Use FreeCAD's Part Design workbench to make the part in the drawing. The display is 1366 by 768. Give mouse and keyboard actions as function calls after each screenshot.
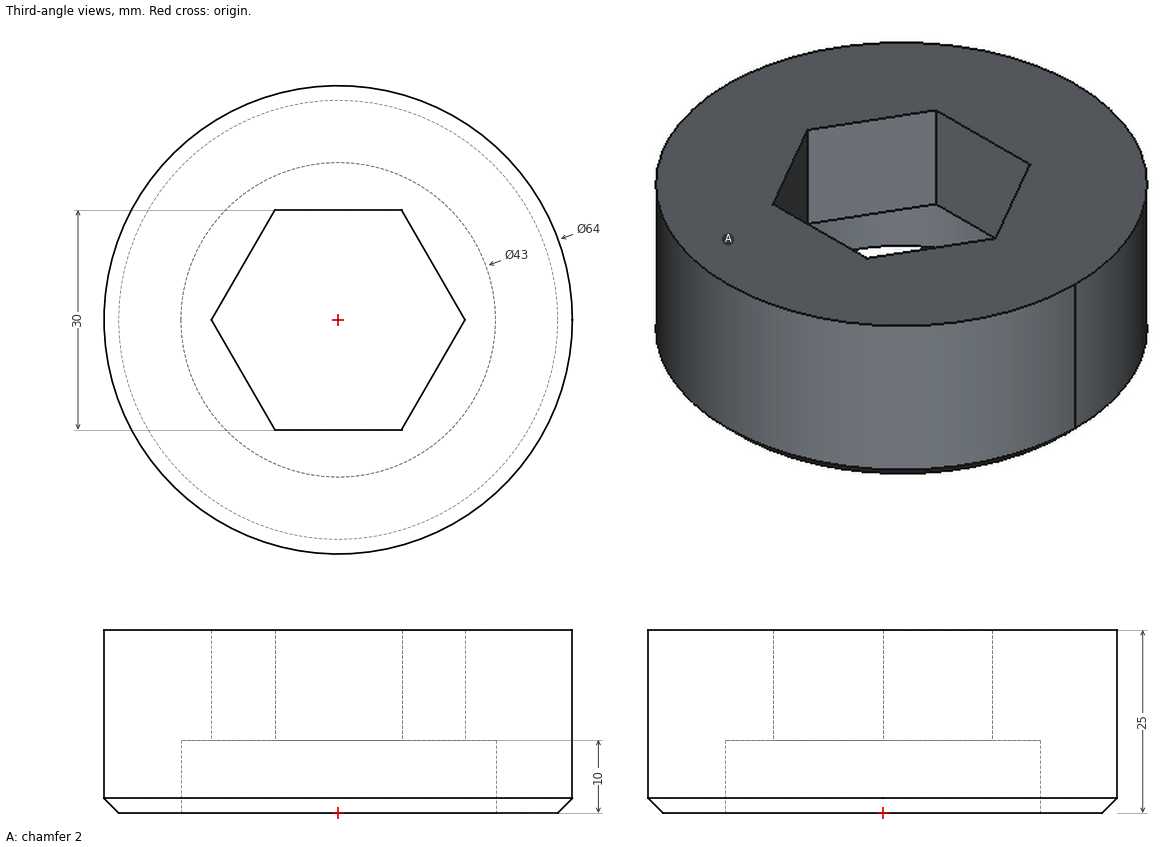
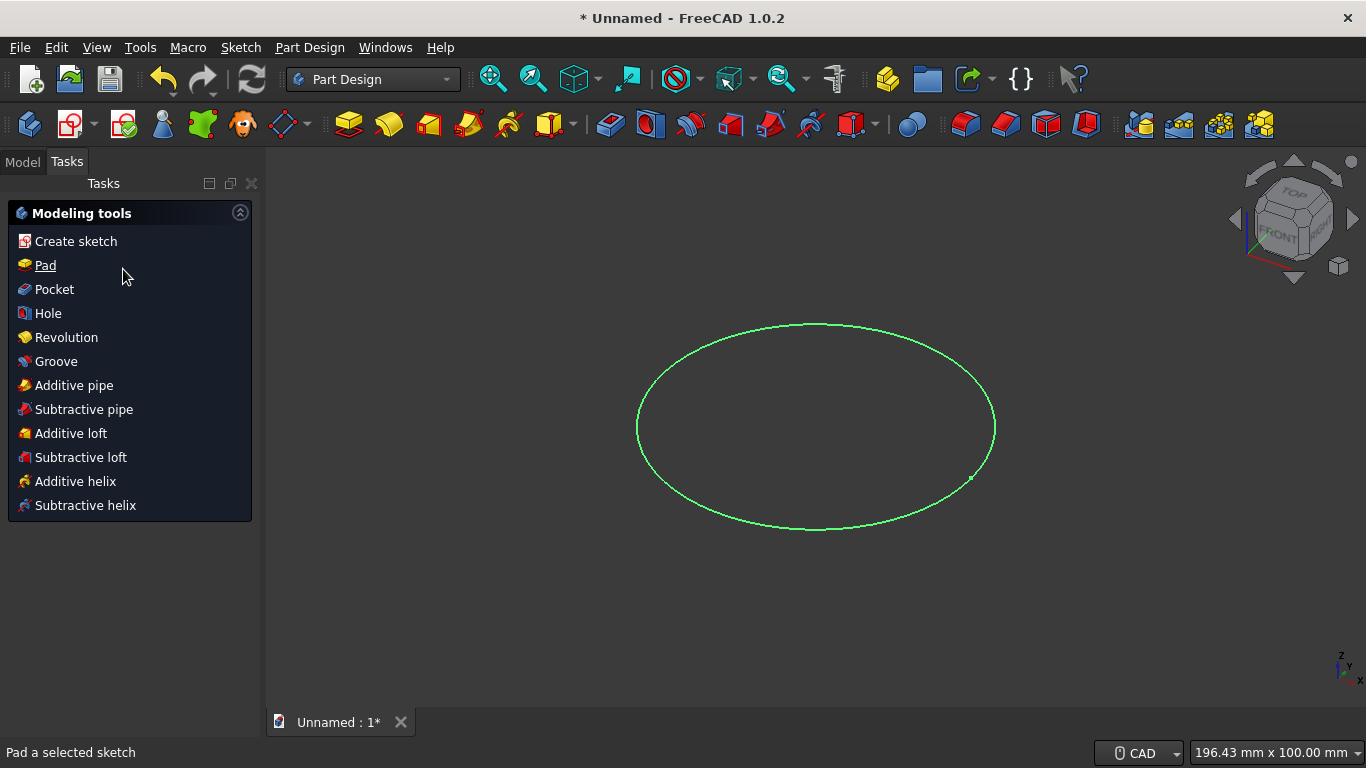
click(350, 124)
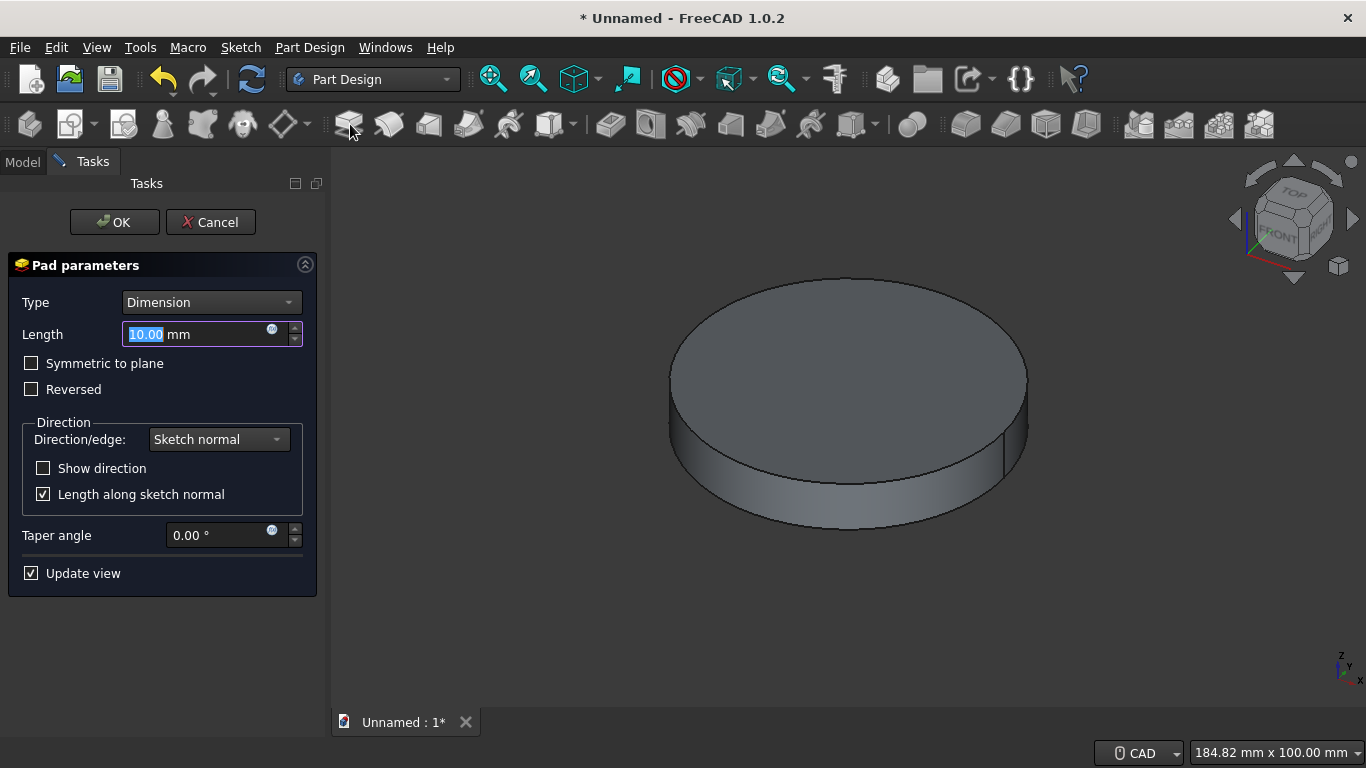
text(25)
key(Tab)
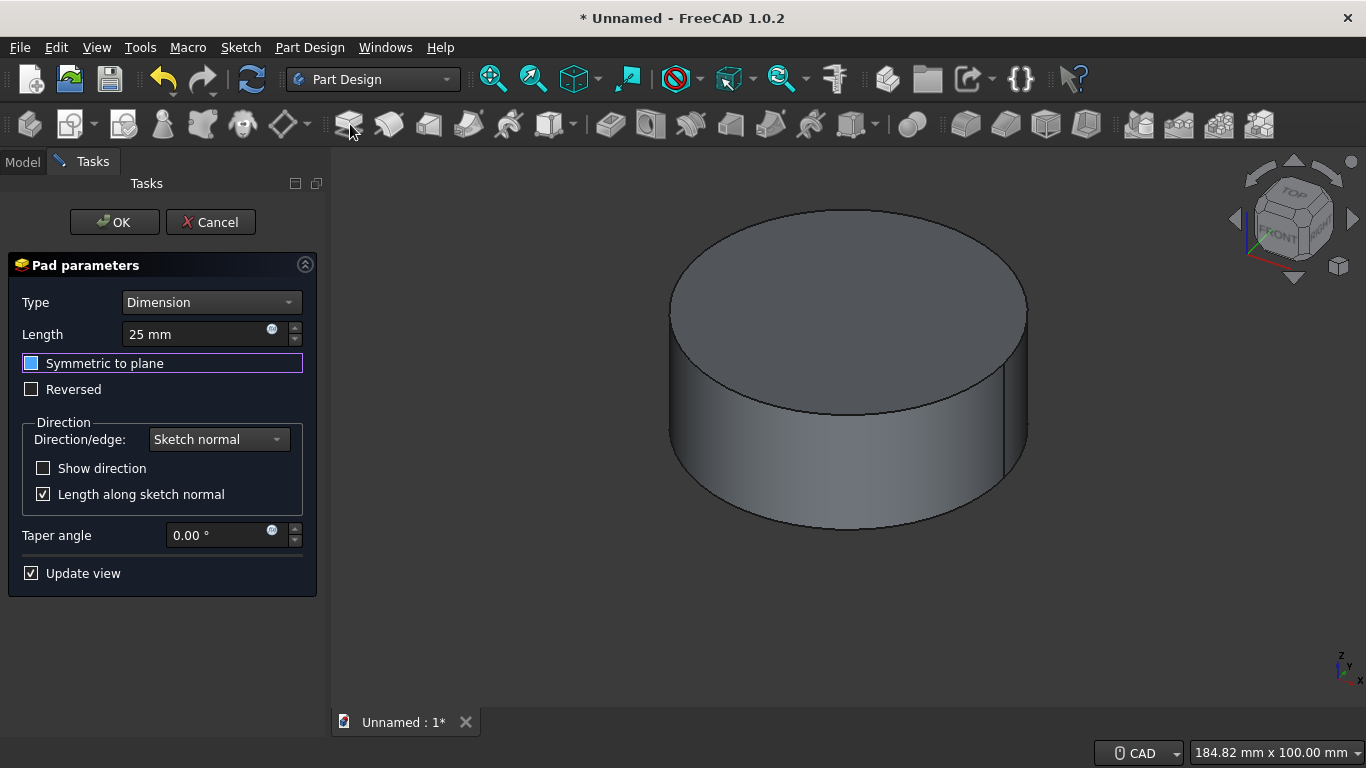
click(115, 222)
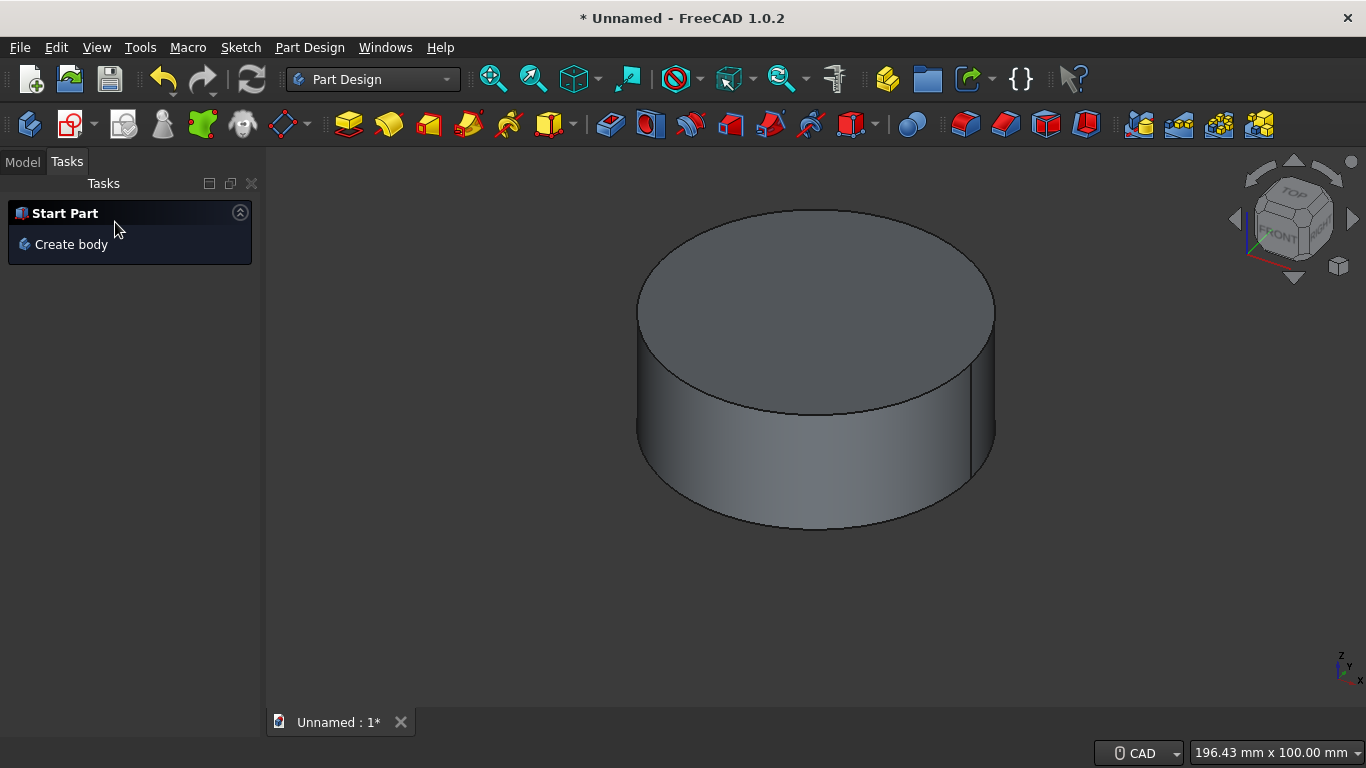
click(816, 311)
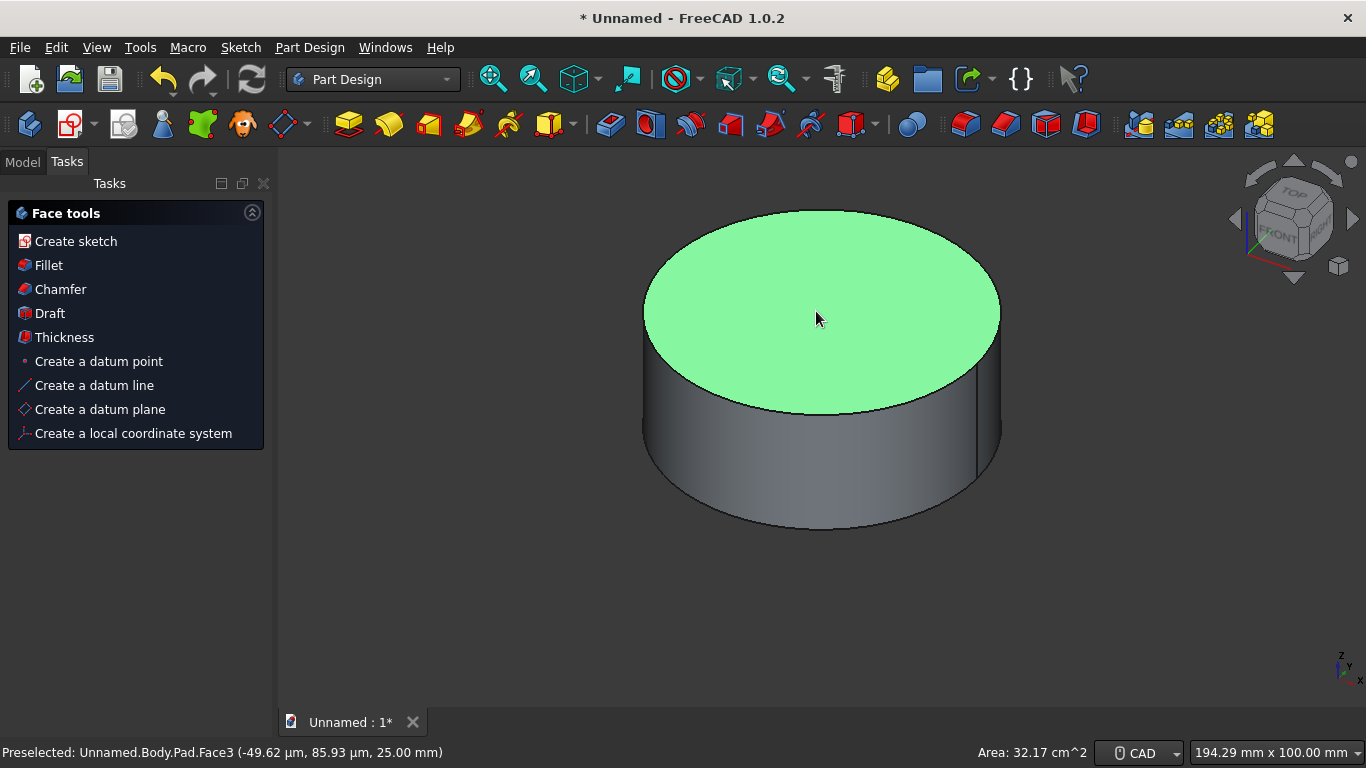
click(70, 124)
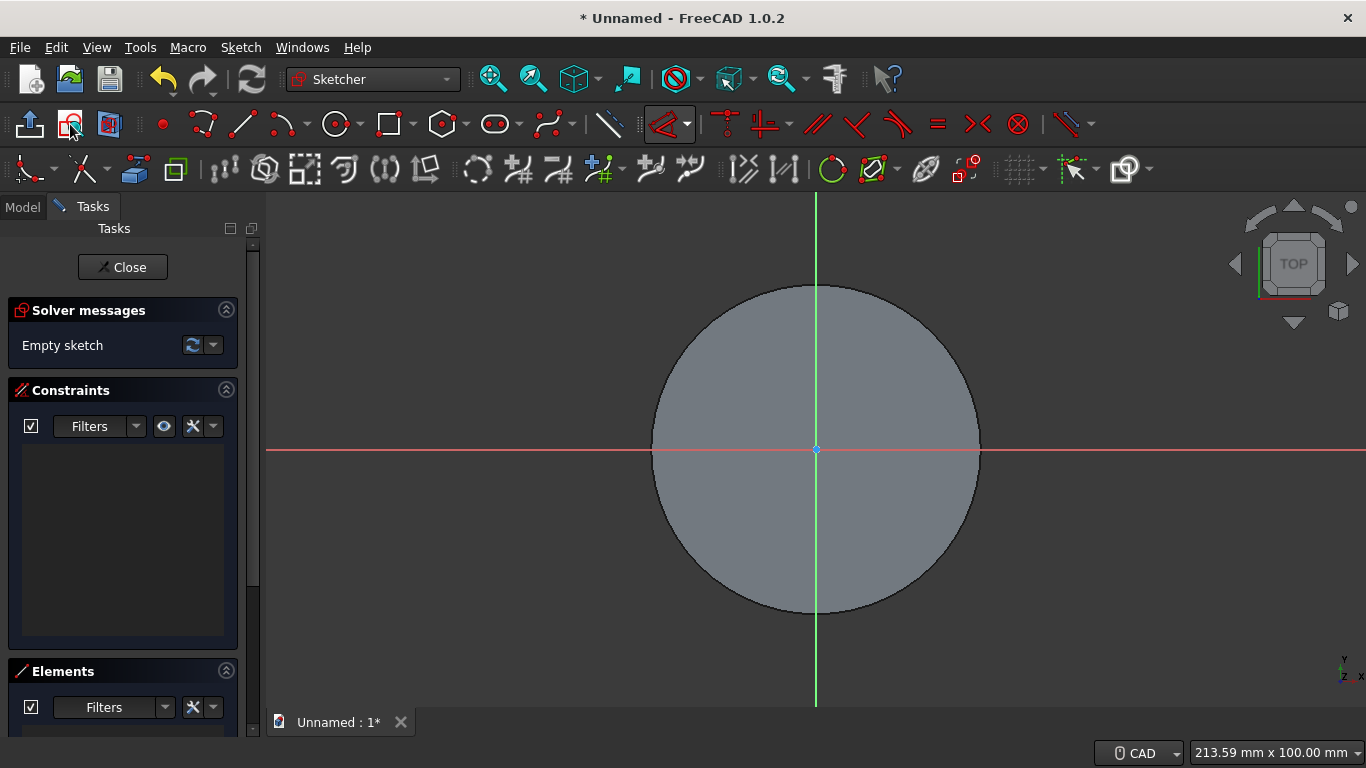
scroll(872, 450, up, 4)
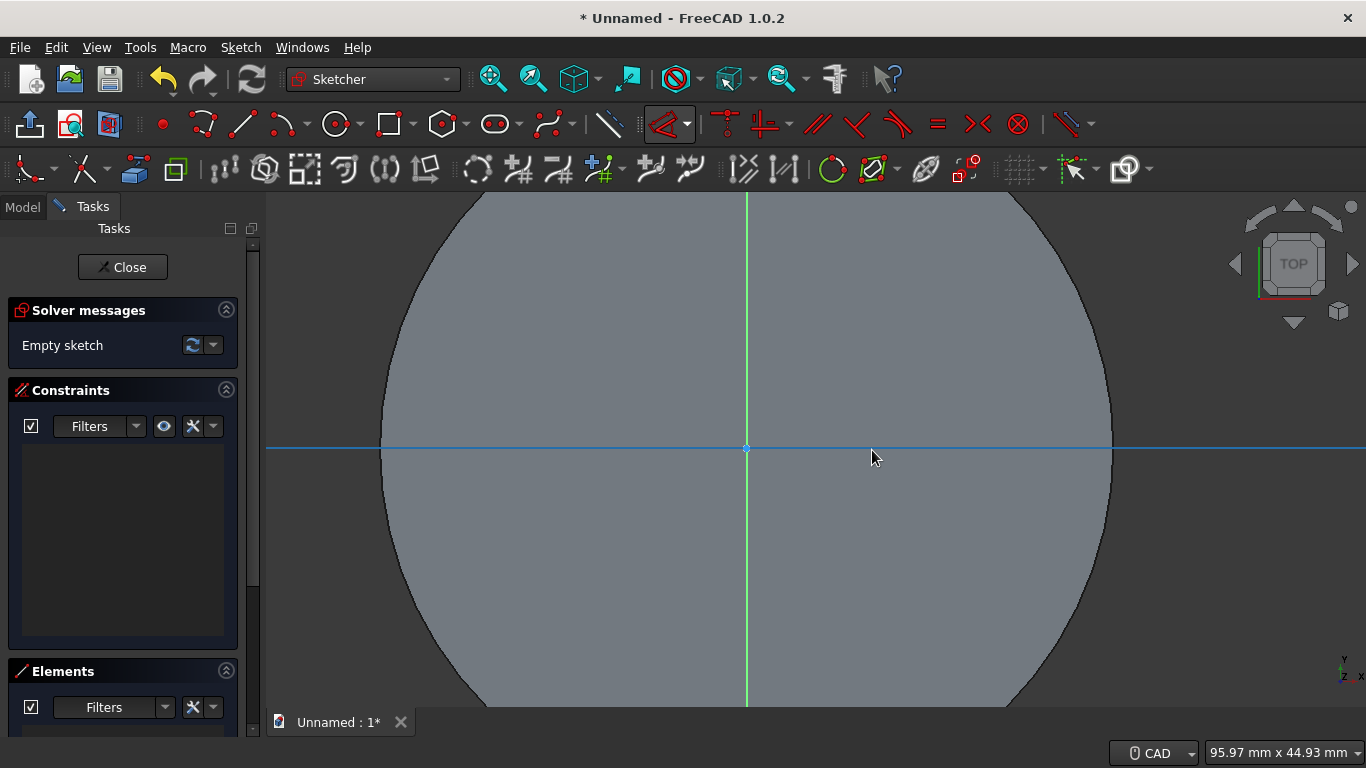
click(442, 124)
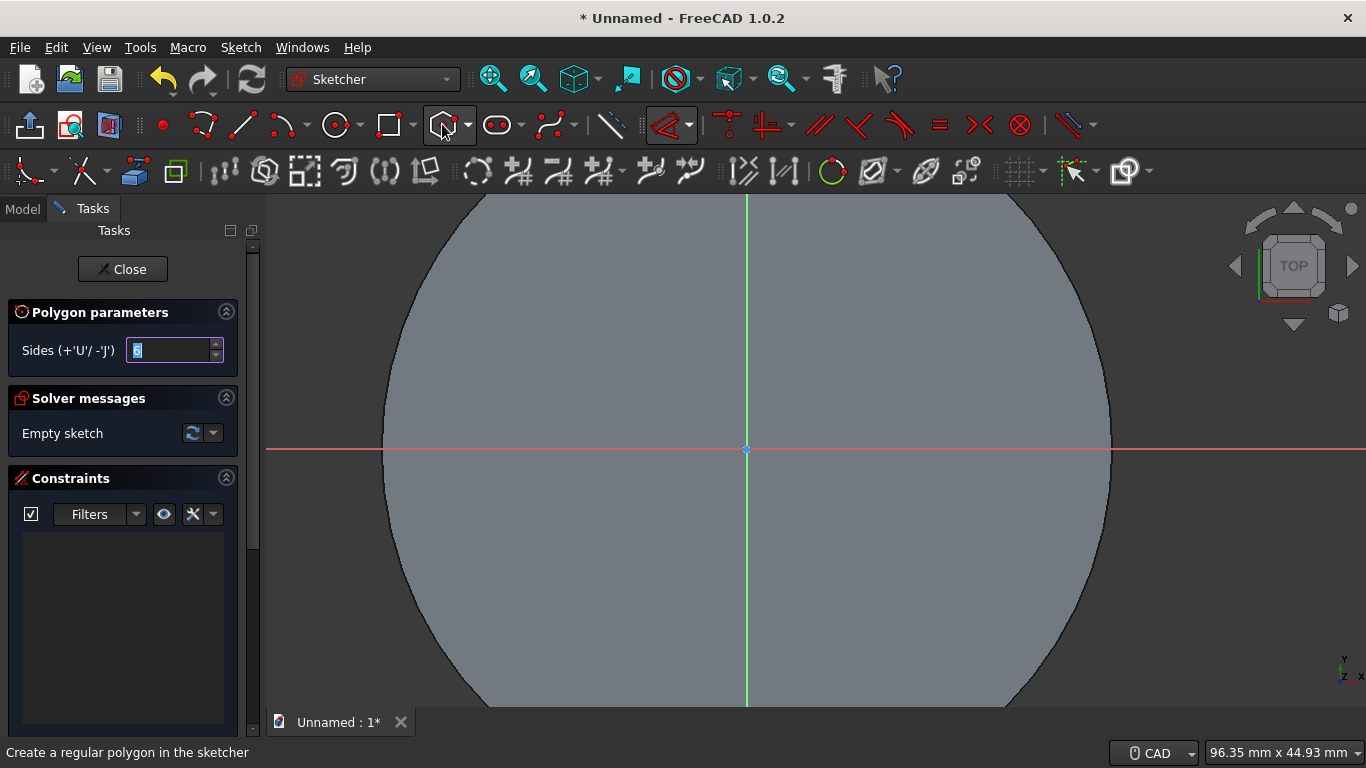
click(747, 449)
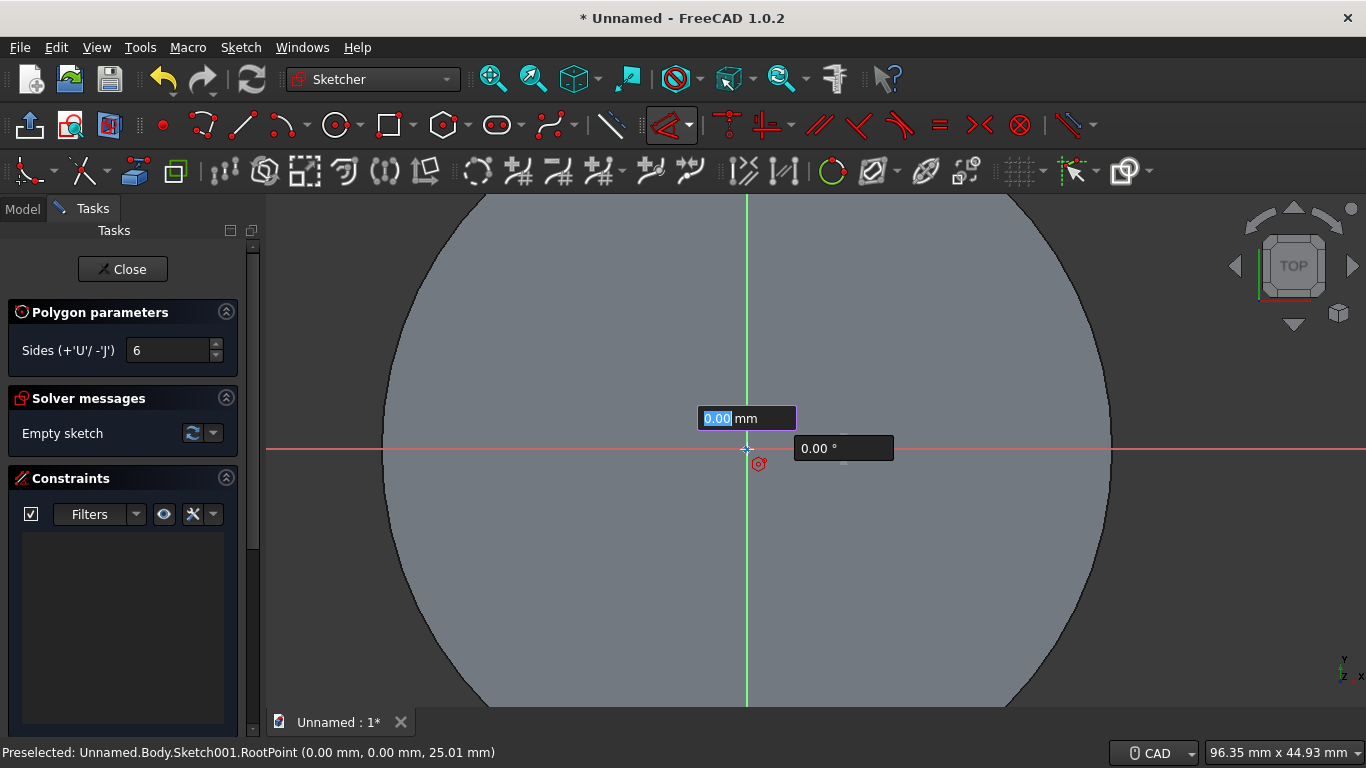
click(945, 449)
right_click(945, 449)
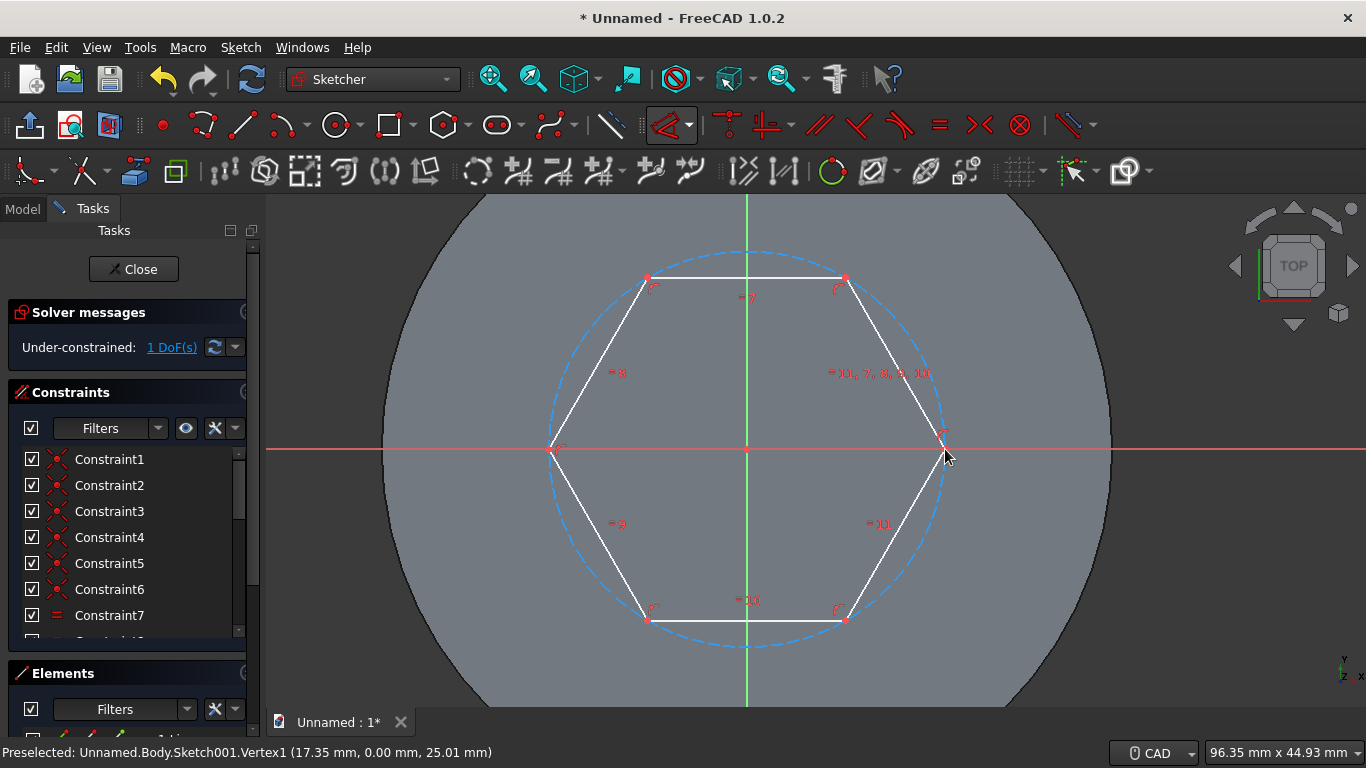
click(666, 126)